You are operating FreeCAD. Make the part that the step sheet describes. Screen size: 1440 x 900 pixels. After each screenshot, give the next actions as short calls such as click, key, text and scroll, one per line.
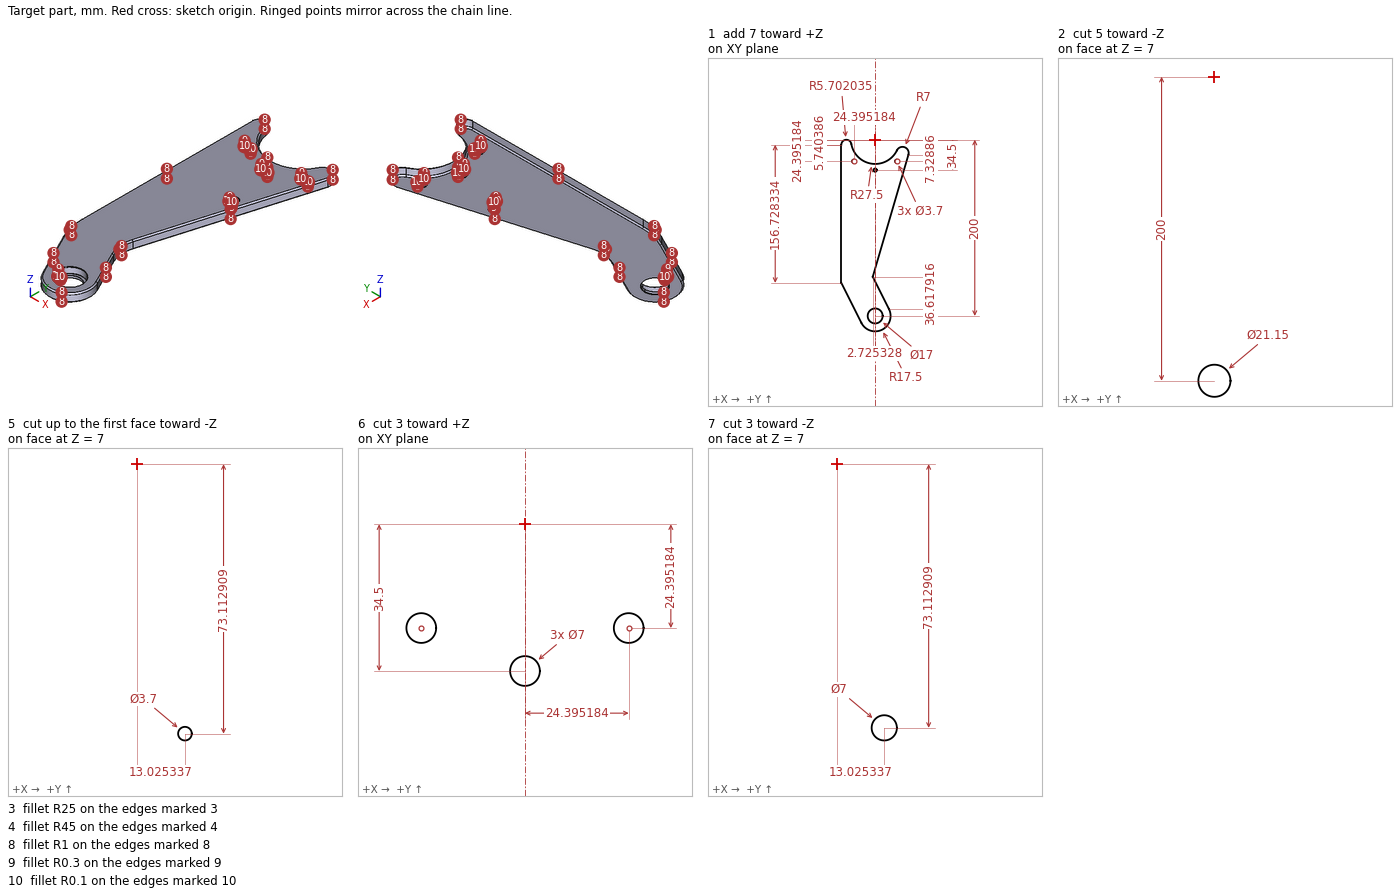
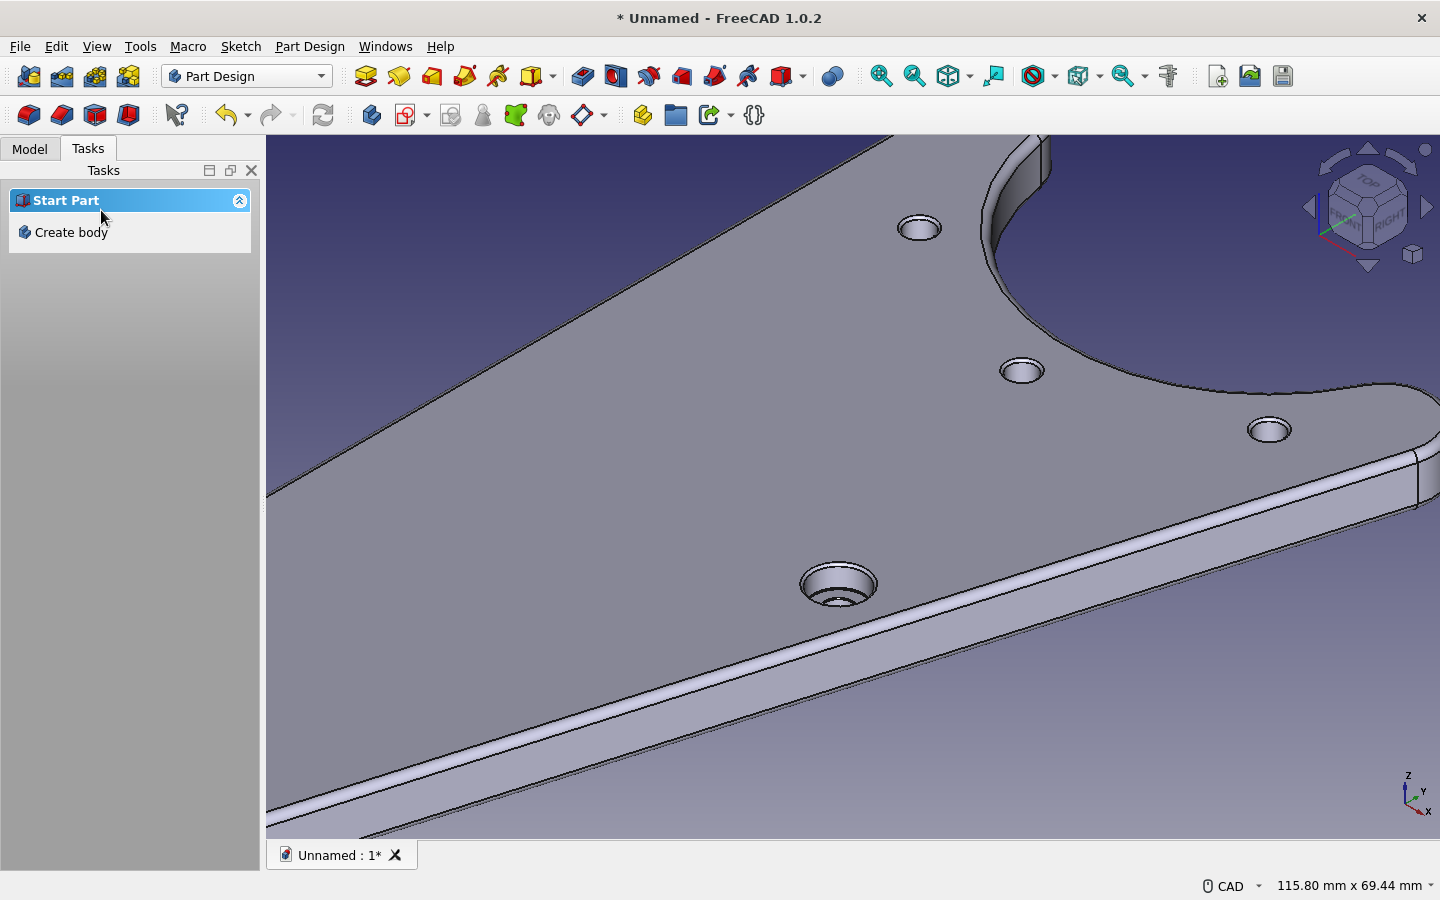
key(v)
key(f)